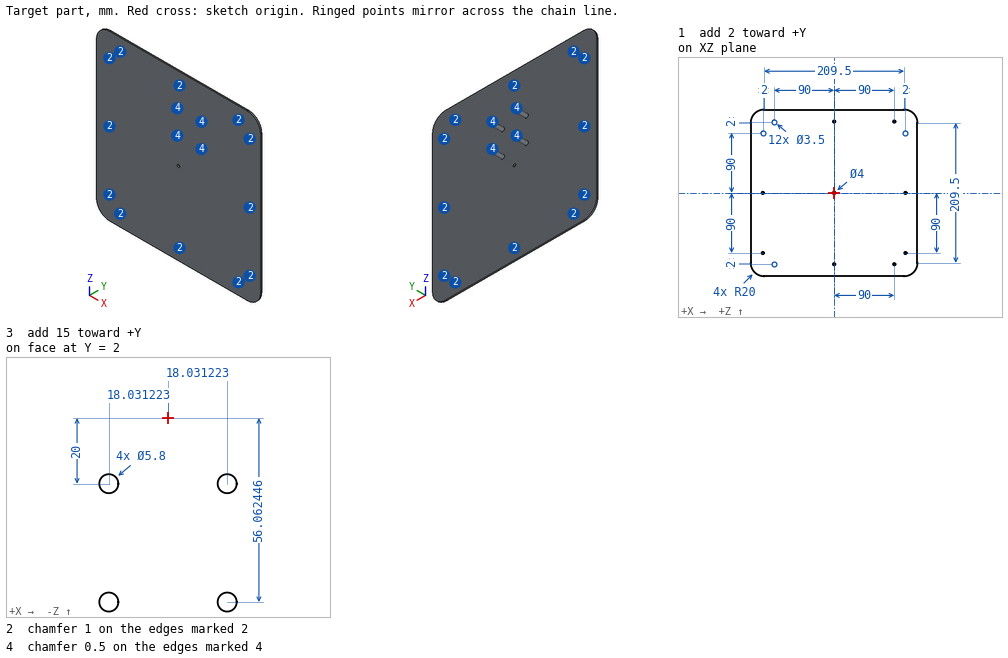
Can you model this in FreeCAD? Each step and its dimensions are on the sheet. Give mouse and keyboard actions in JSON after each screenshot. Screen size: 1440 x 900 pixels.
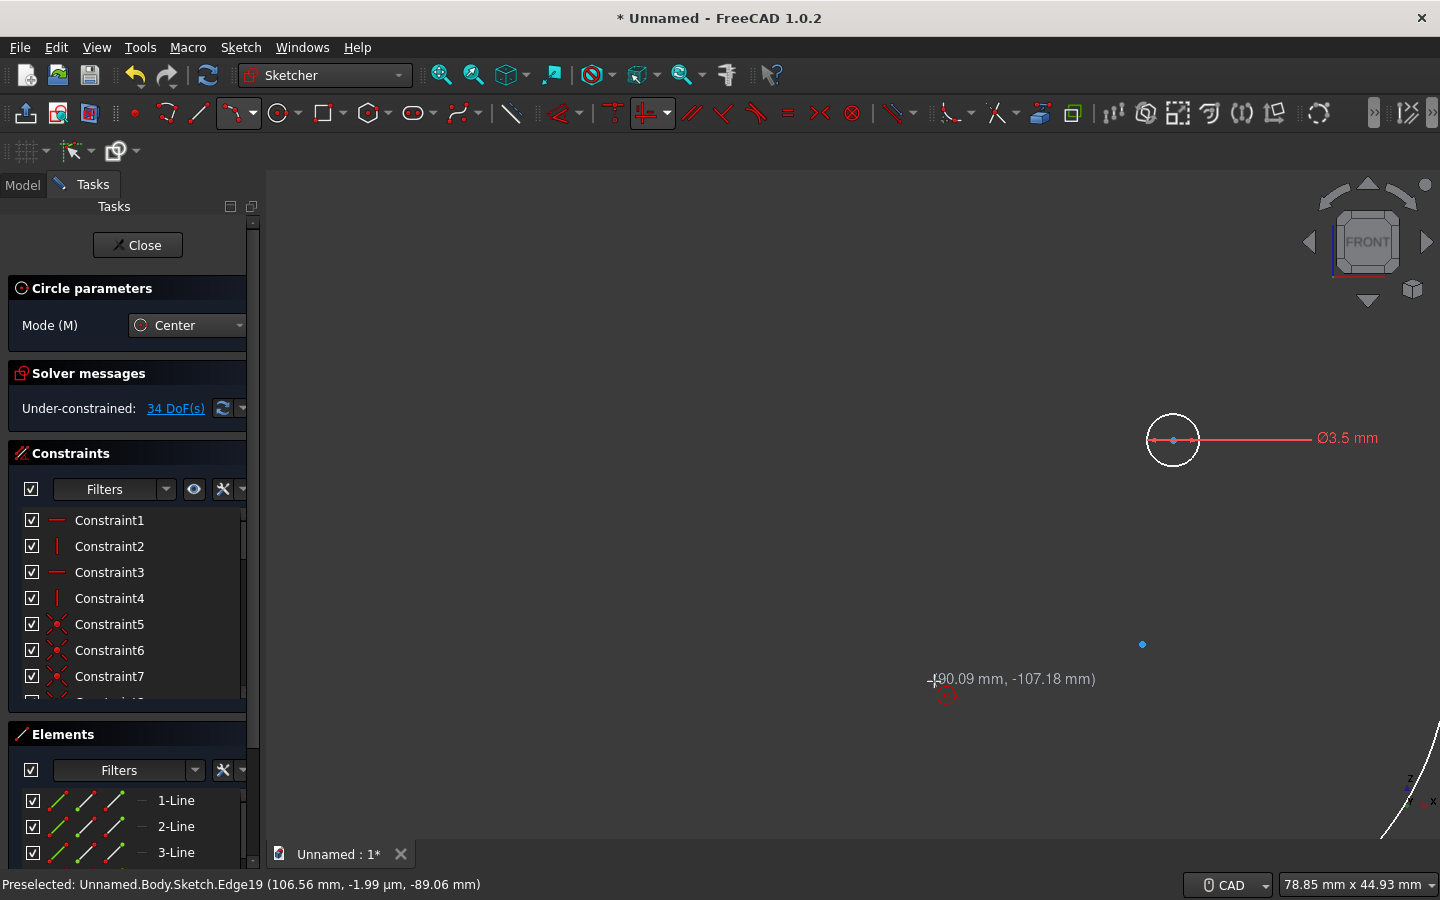
{"action": "scroll", "coordinate": [934, 681], "scroll_direction": "down", "scroll_amount": 11}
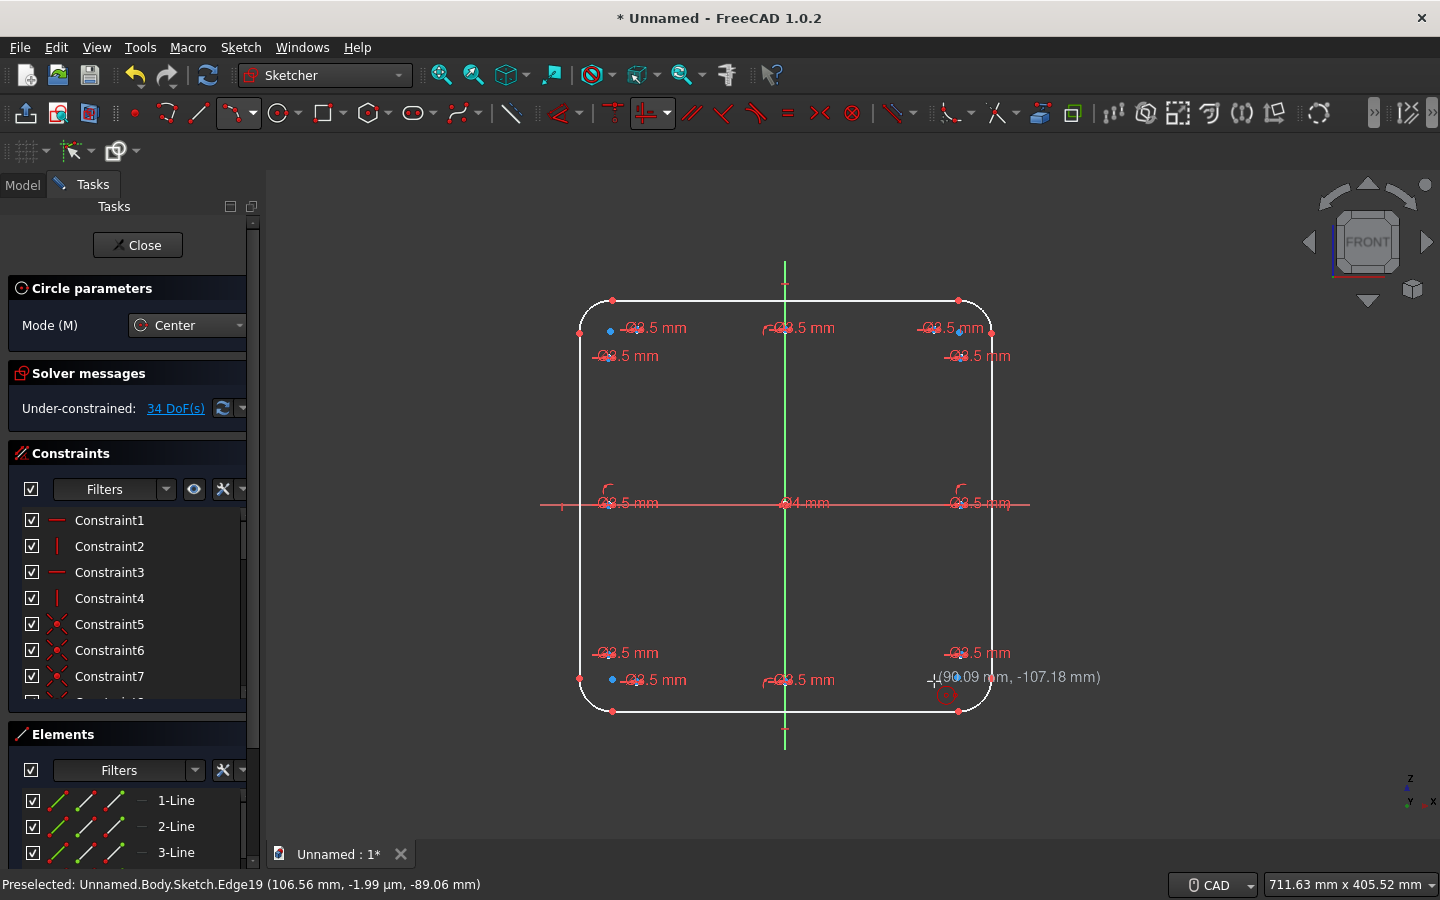
{"action": "left_click", "coordinate": [934, 681]}
{"action": "mouse_move", "coordinate": [936, 679]}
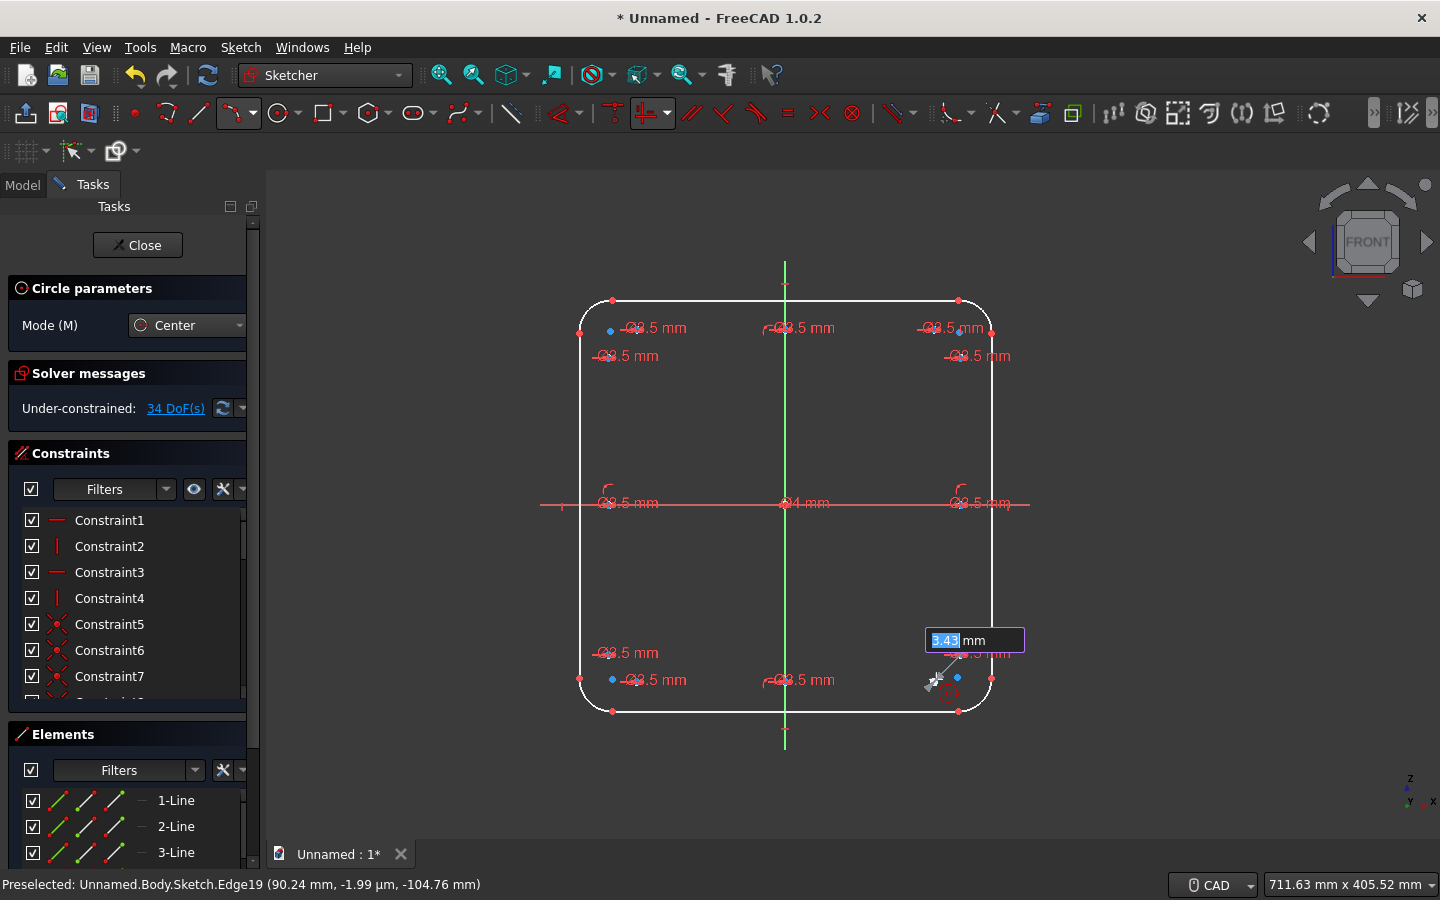
{"action": "type", "text": "3.5"}
{"action": "key", "text": "Return"}
{"action": "key", "text": "Escape"}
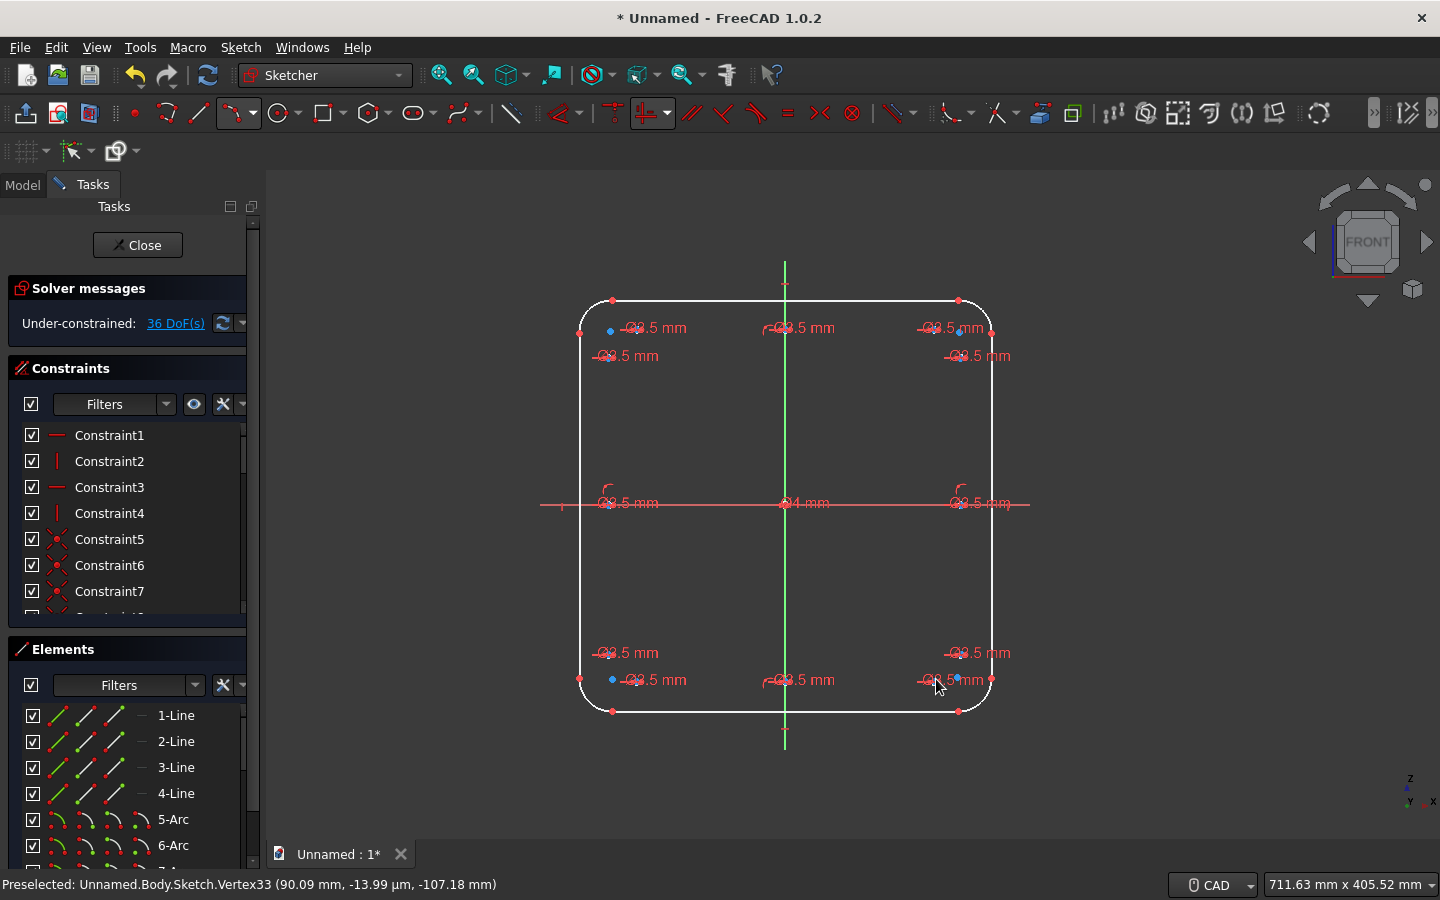
{"action": "left_click", "coordinate": [716, 301]}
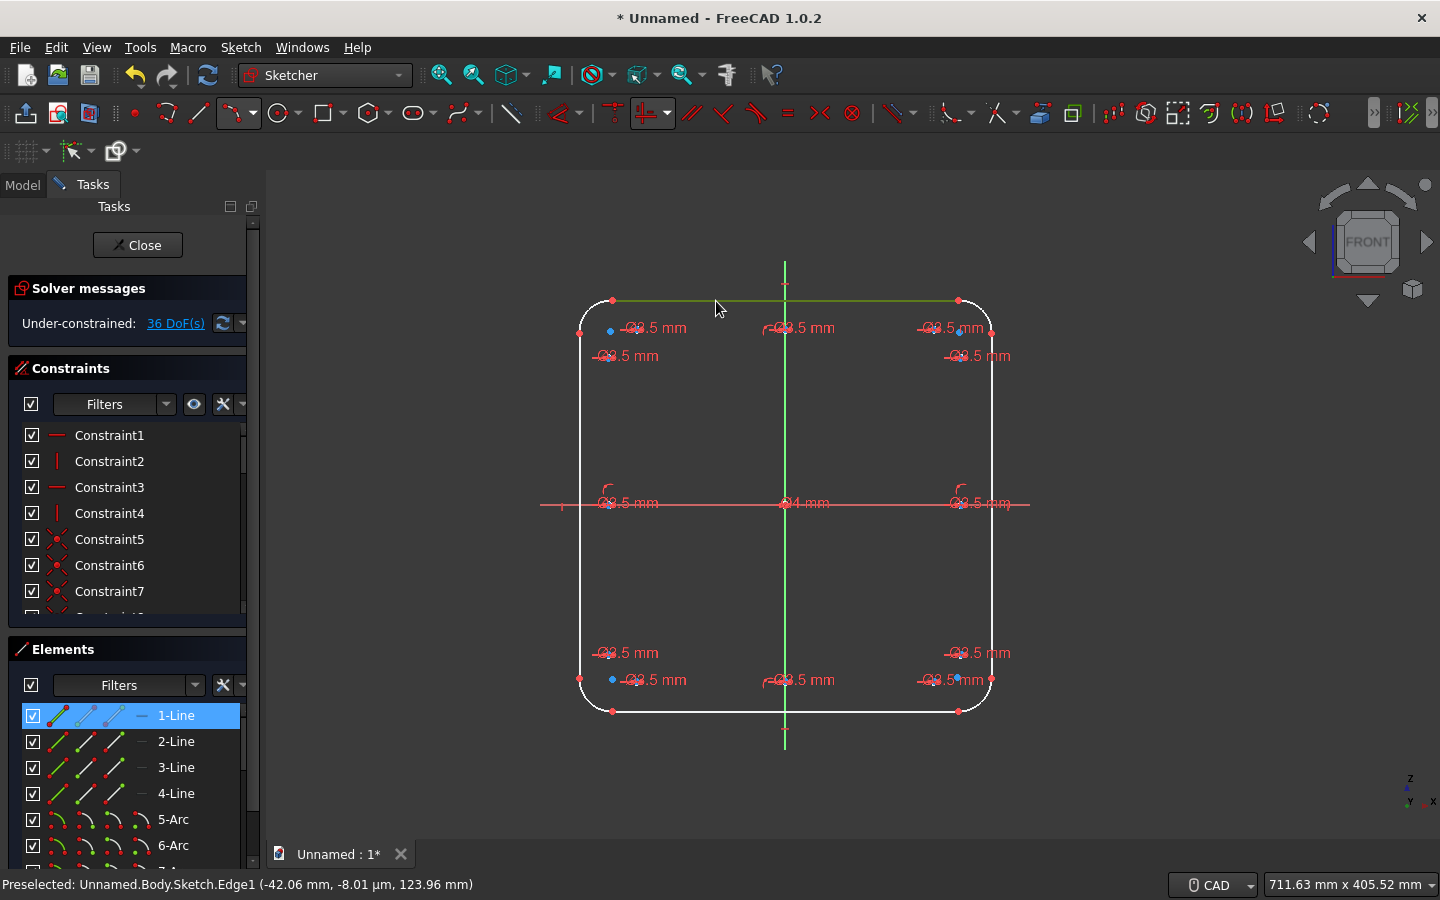
{"action": "left_click", "coordinate": [988, 319]}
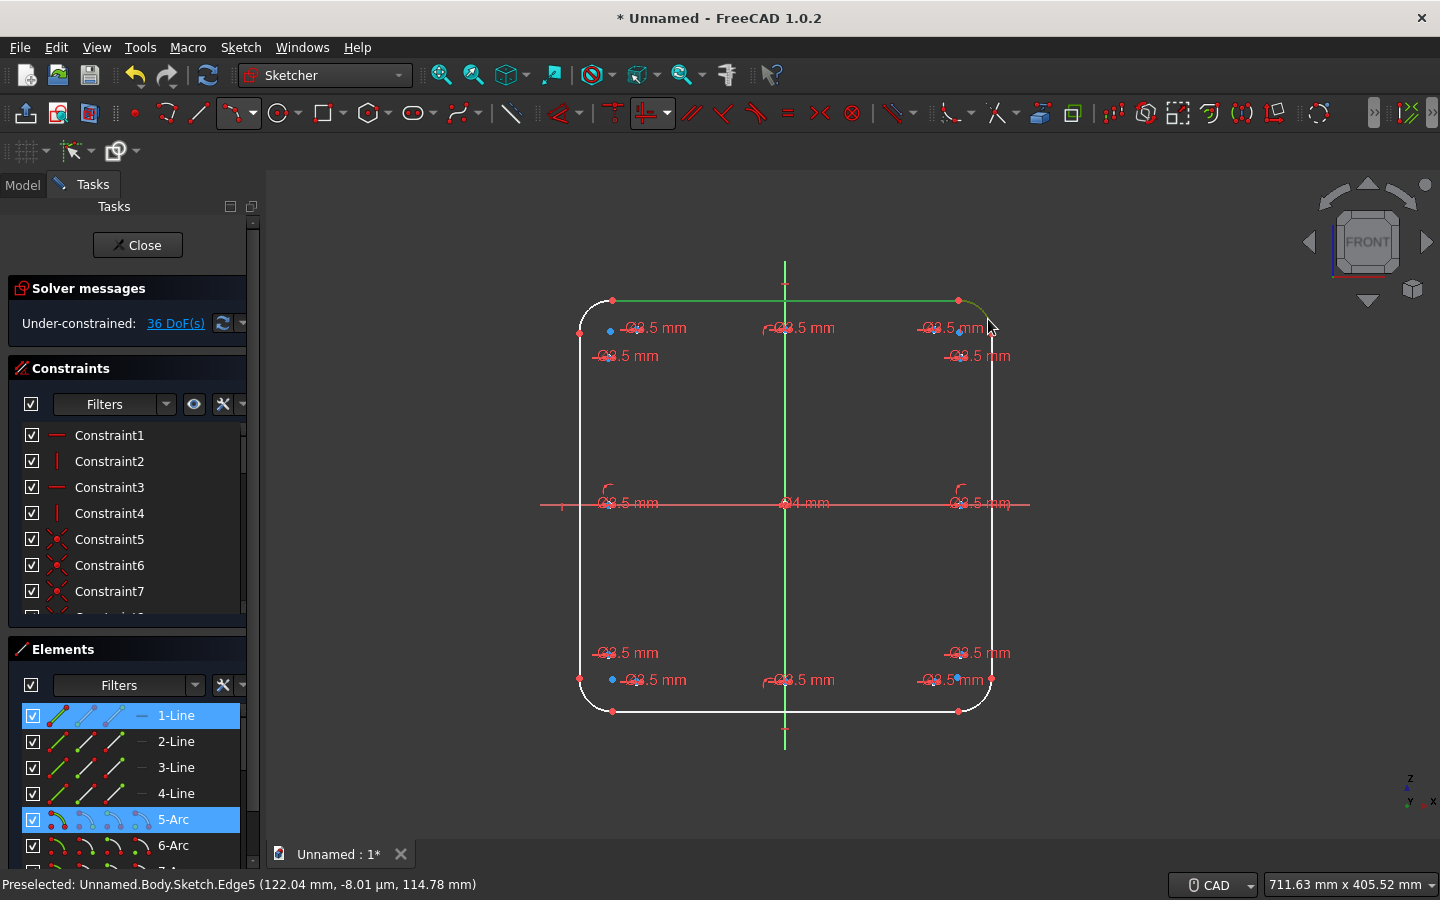
{"action": "left_click", "coordinate": [756, 114]}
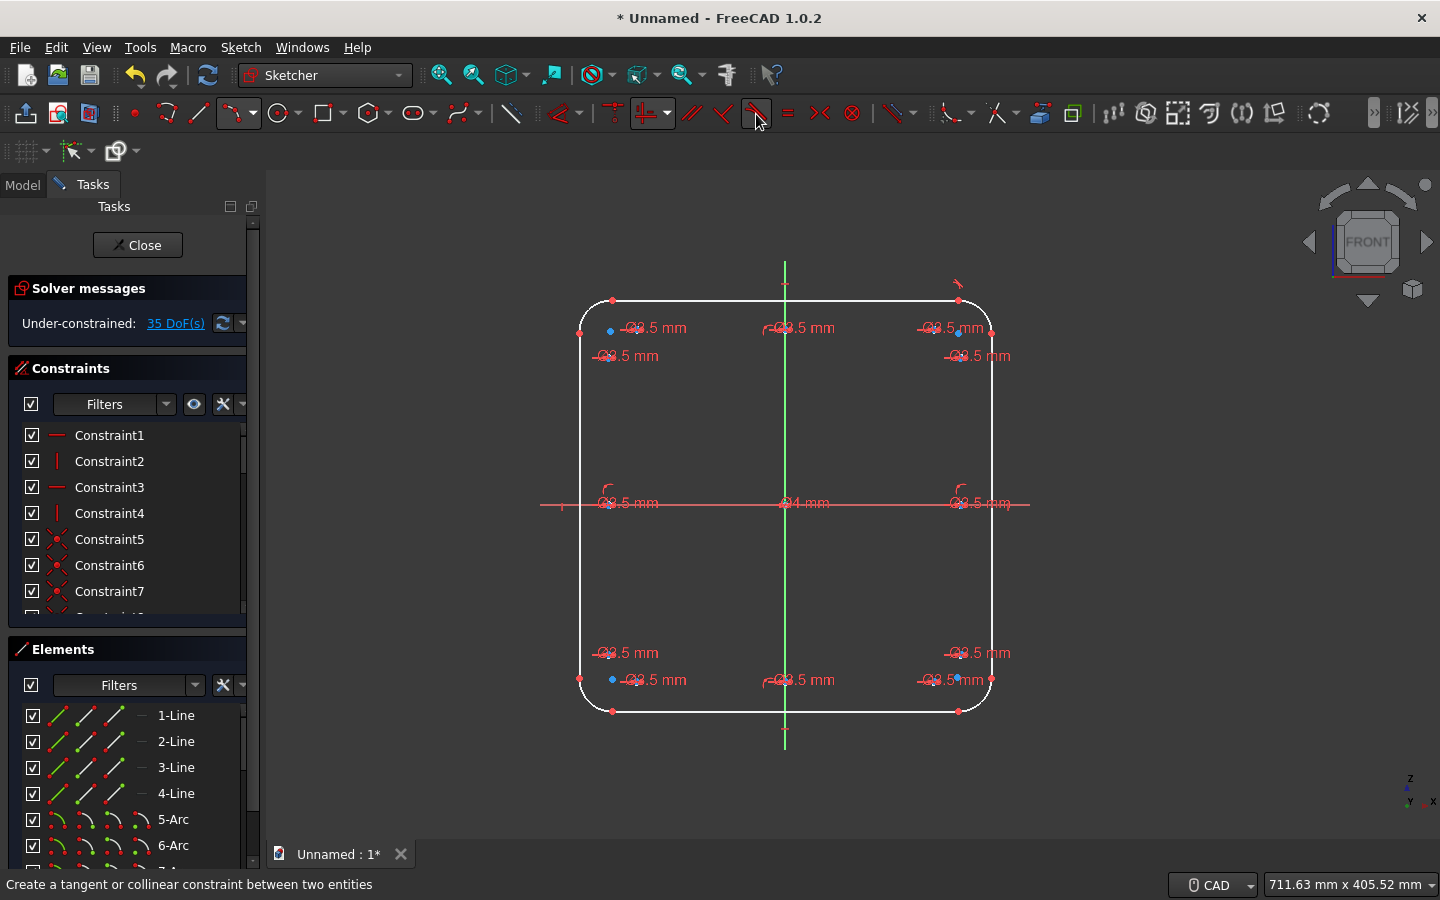
{"action": "left_click", "coordinate": [716, 301]}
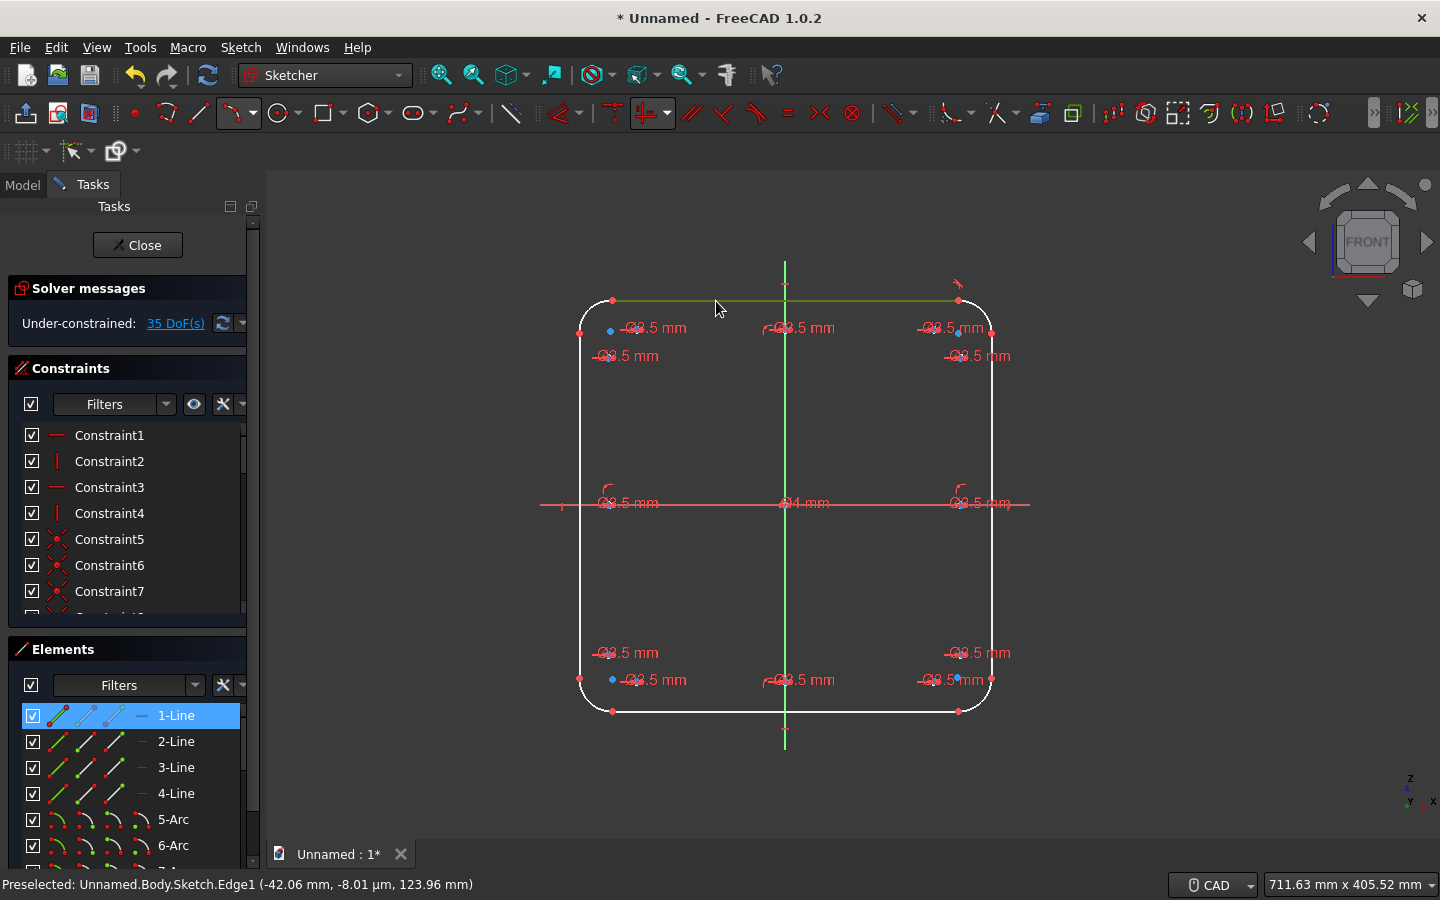
{"action": "left_click", "coordinate": [597, 304]}